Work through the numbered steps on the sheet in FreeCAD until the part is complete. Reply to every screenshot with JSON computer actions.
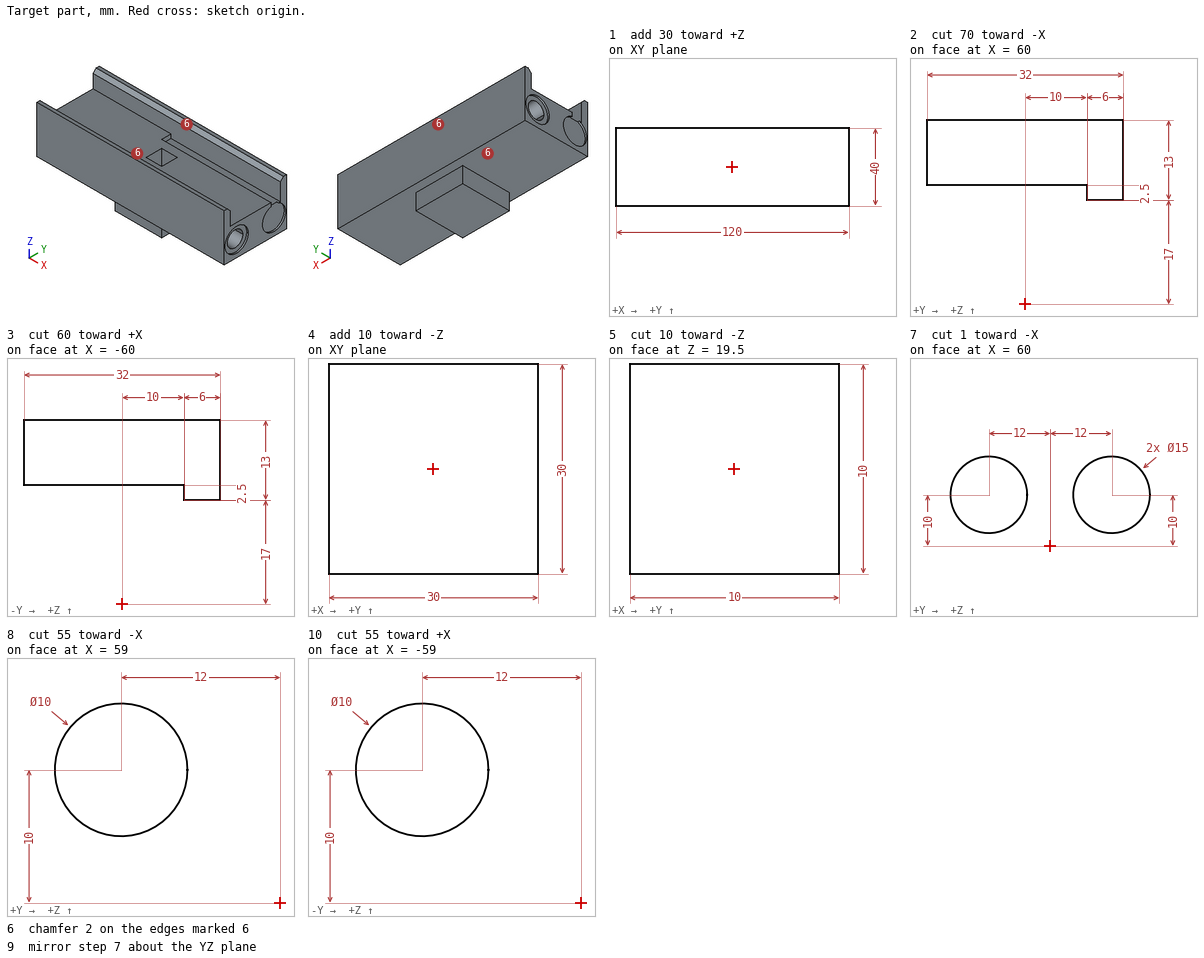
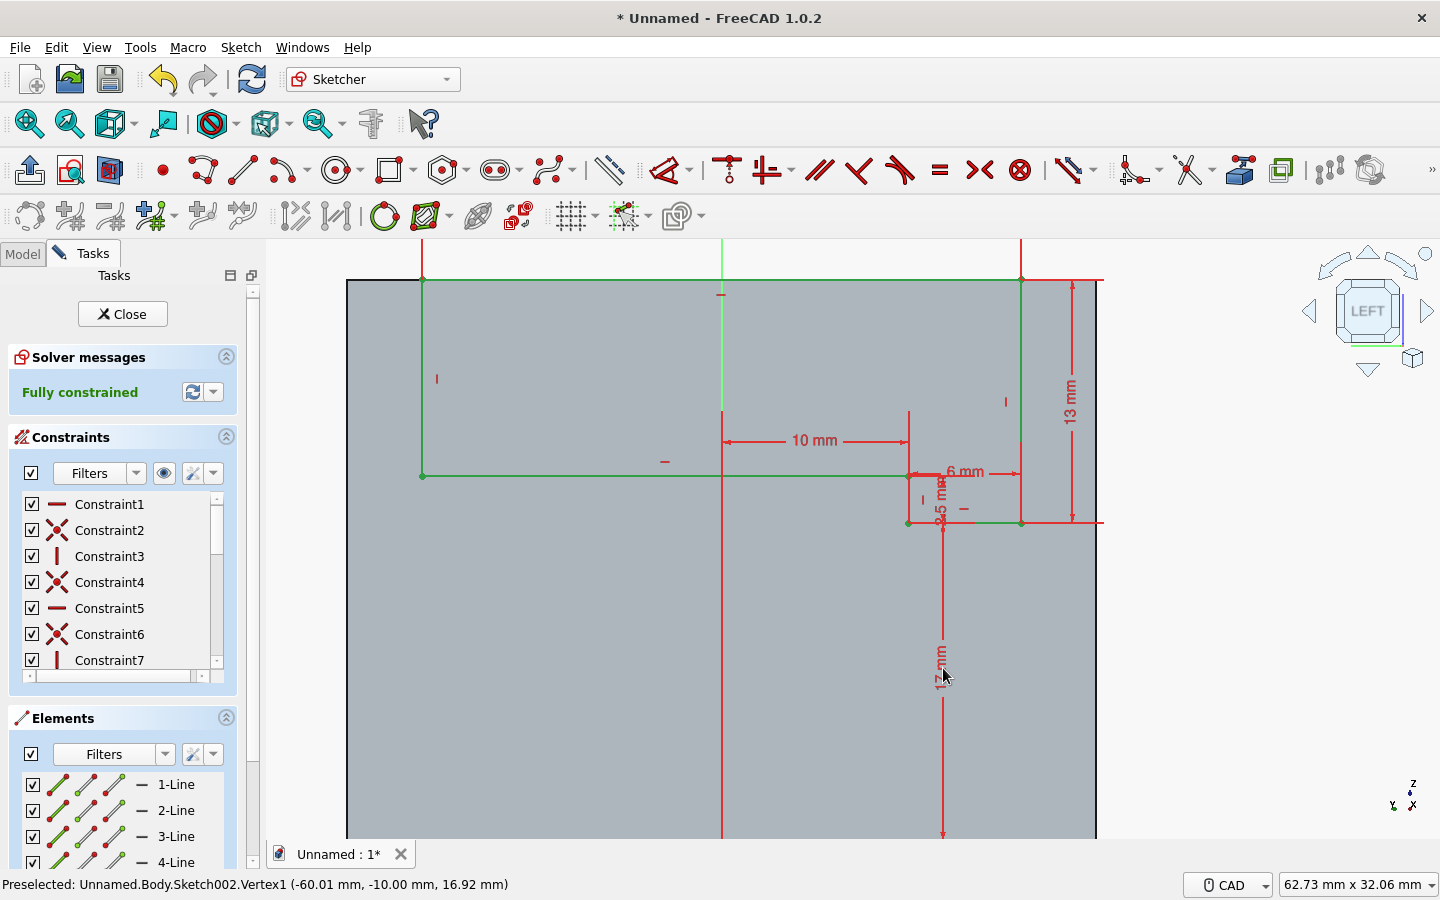
{"action": "left_click", "coordinate": [123, 314]}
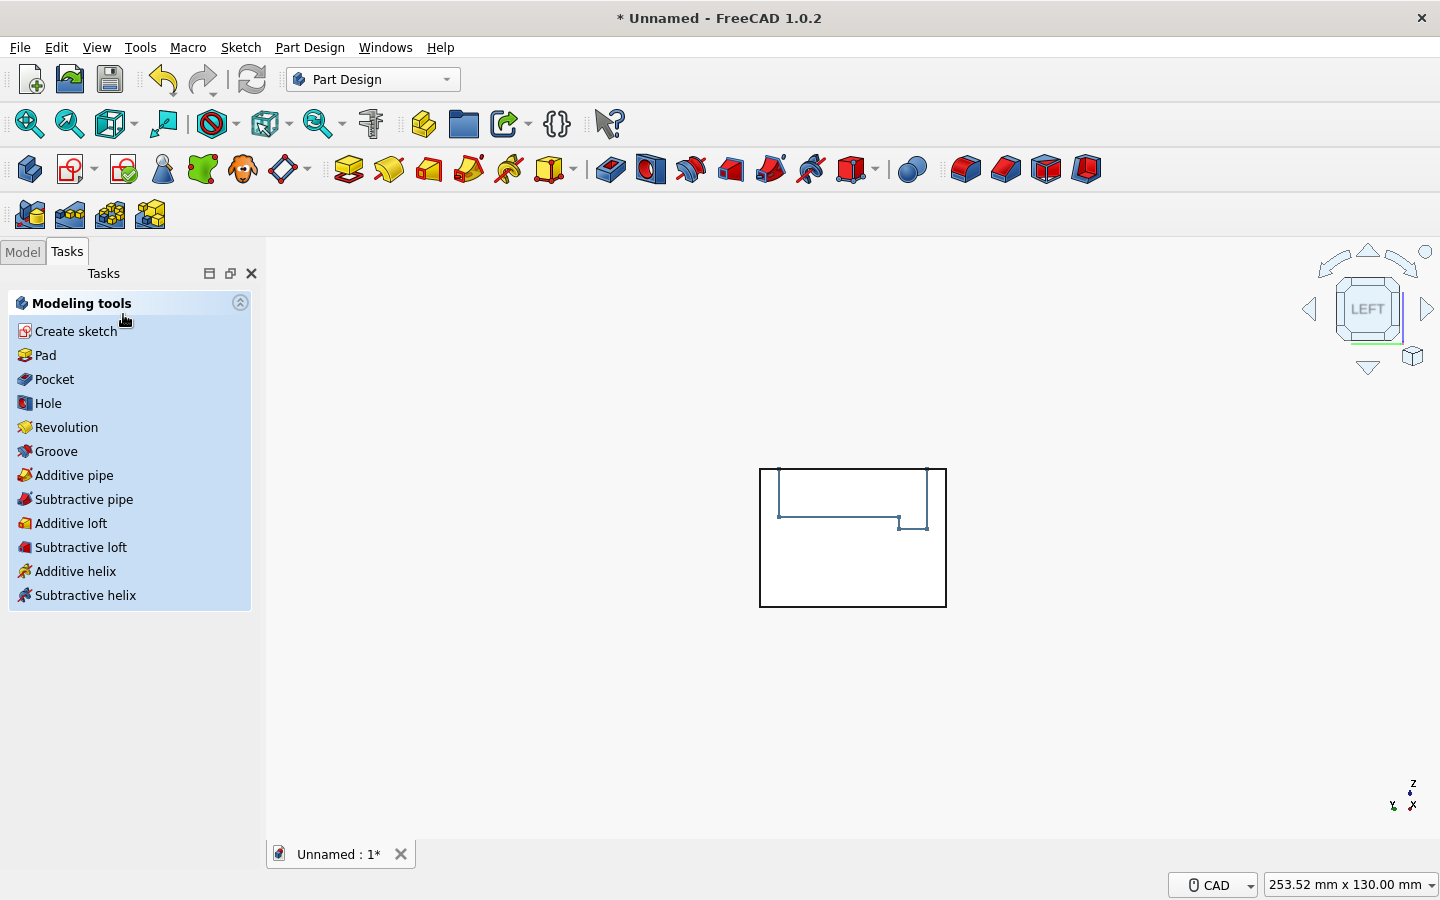
{"action": "left_click", "coordinate": [612, 170]}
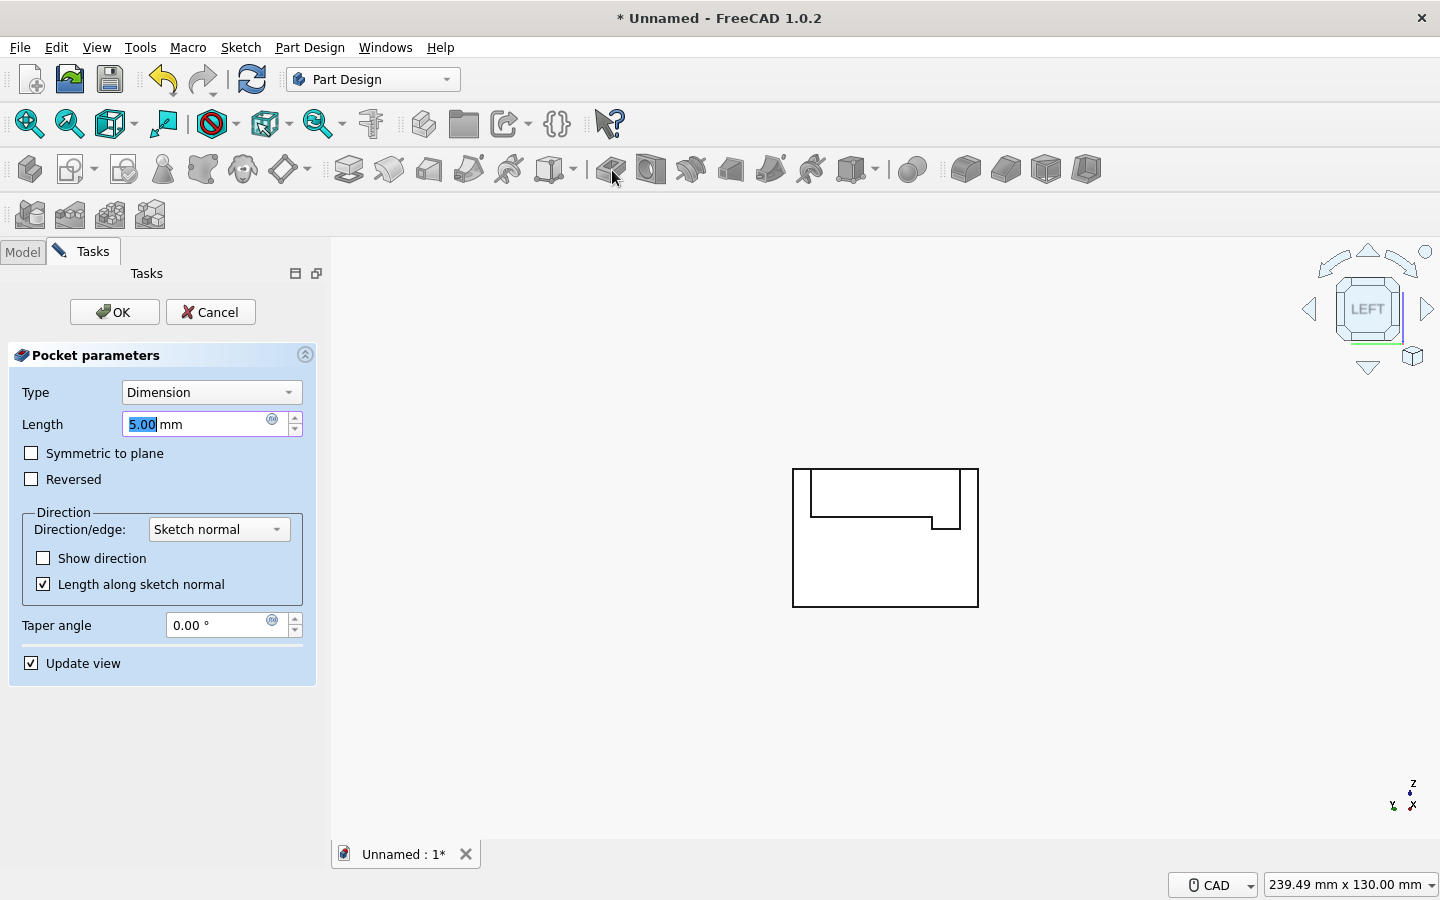
{"action": "type", "text": "60"}
{"action": "key", "text": "Tab"}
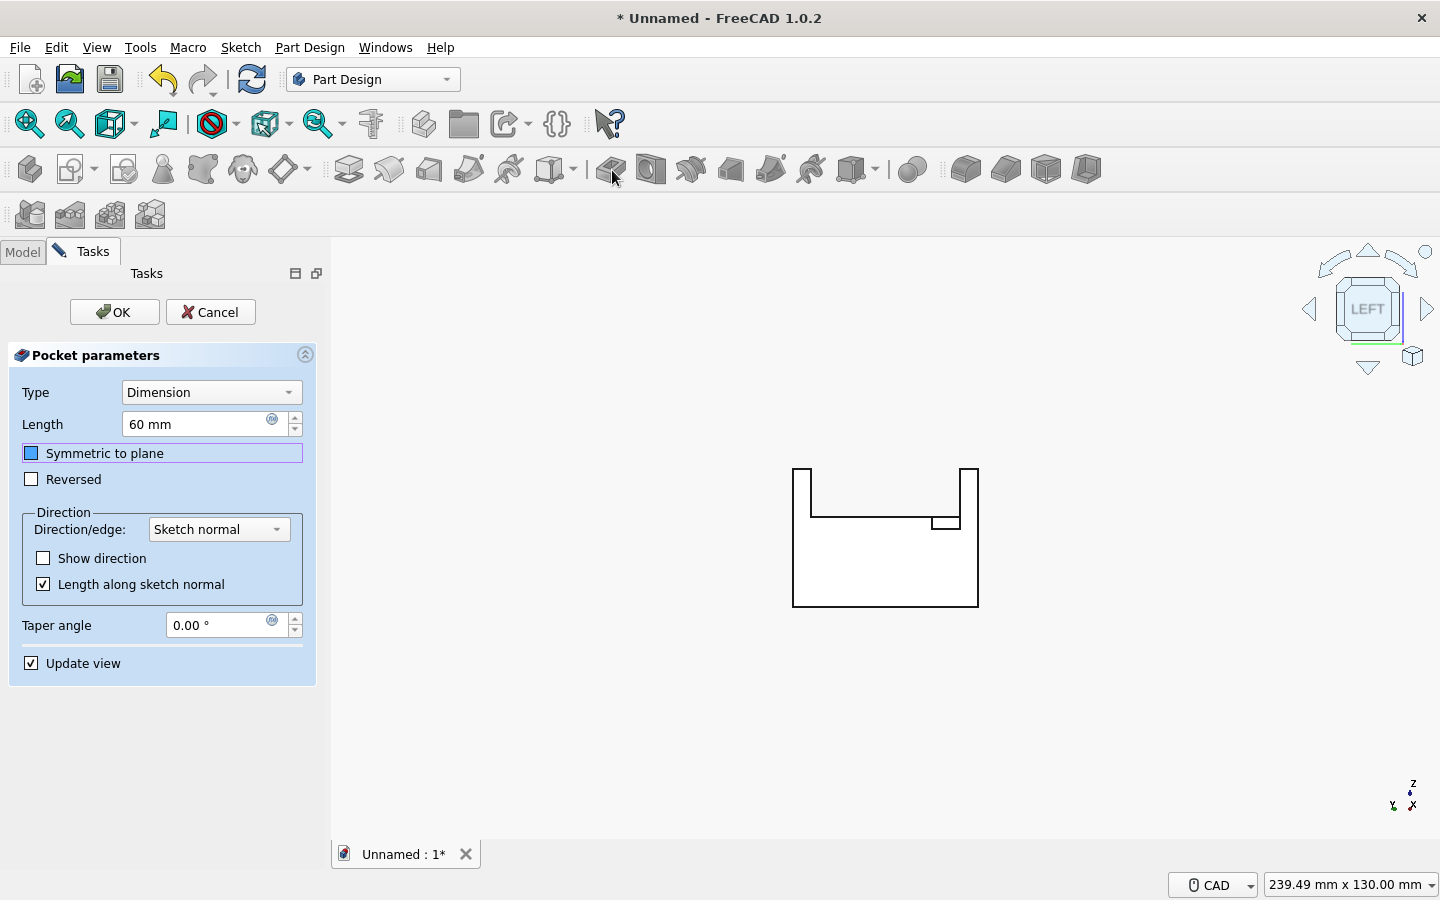
{"action": "left_click", "coordinate": [115, 312]}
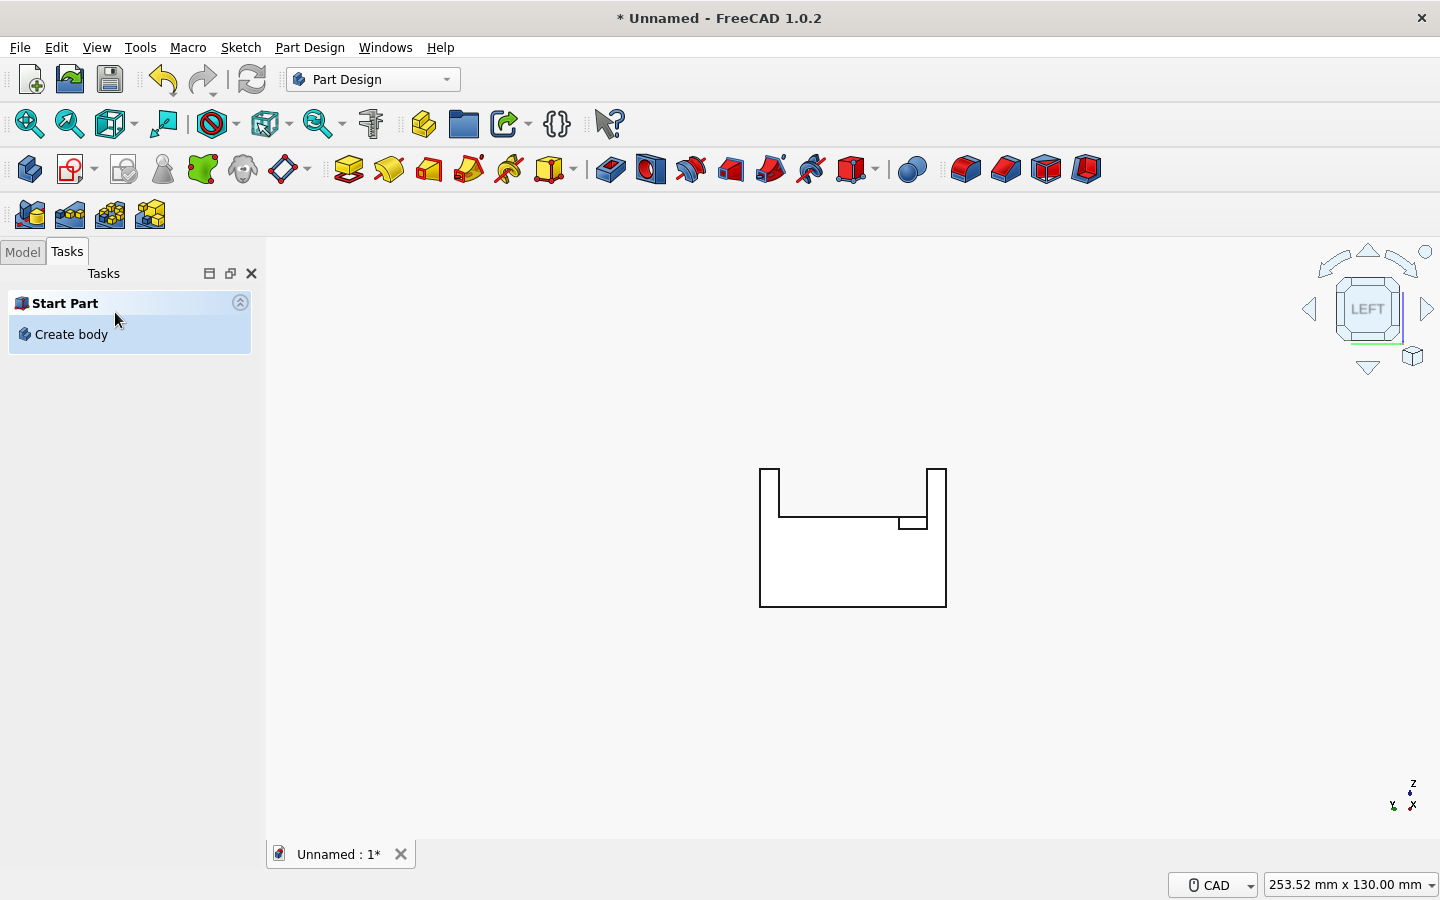
{"action": "left_click", "coordinate": [30, 124]}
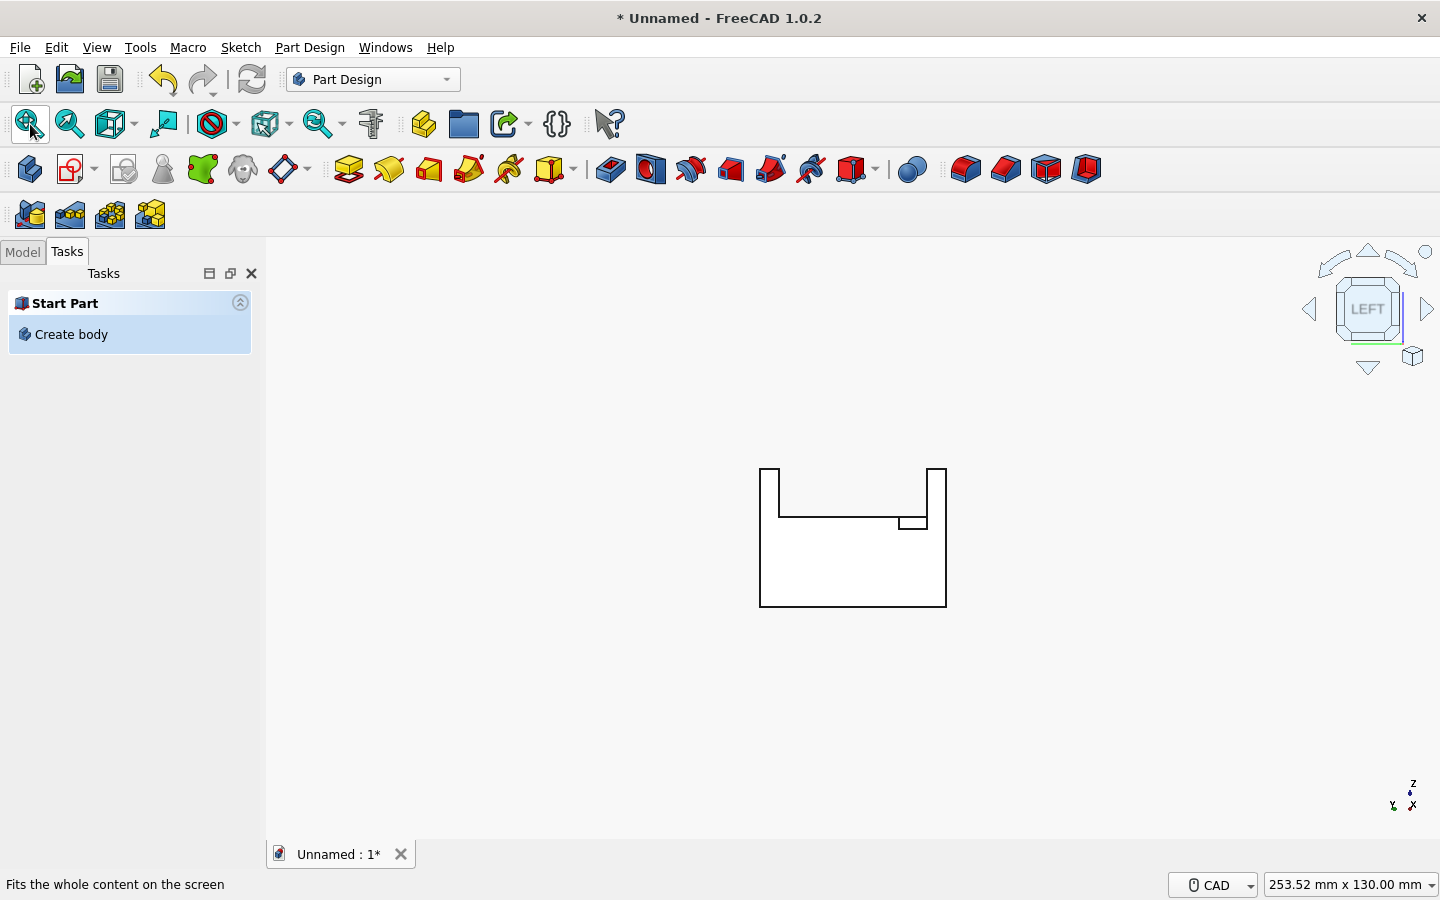
{"action": "left_click", "coordinate": [70, 170]}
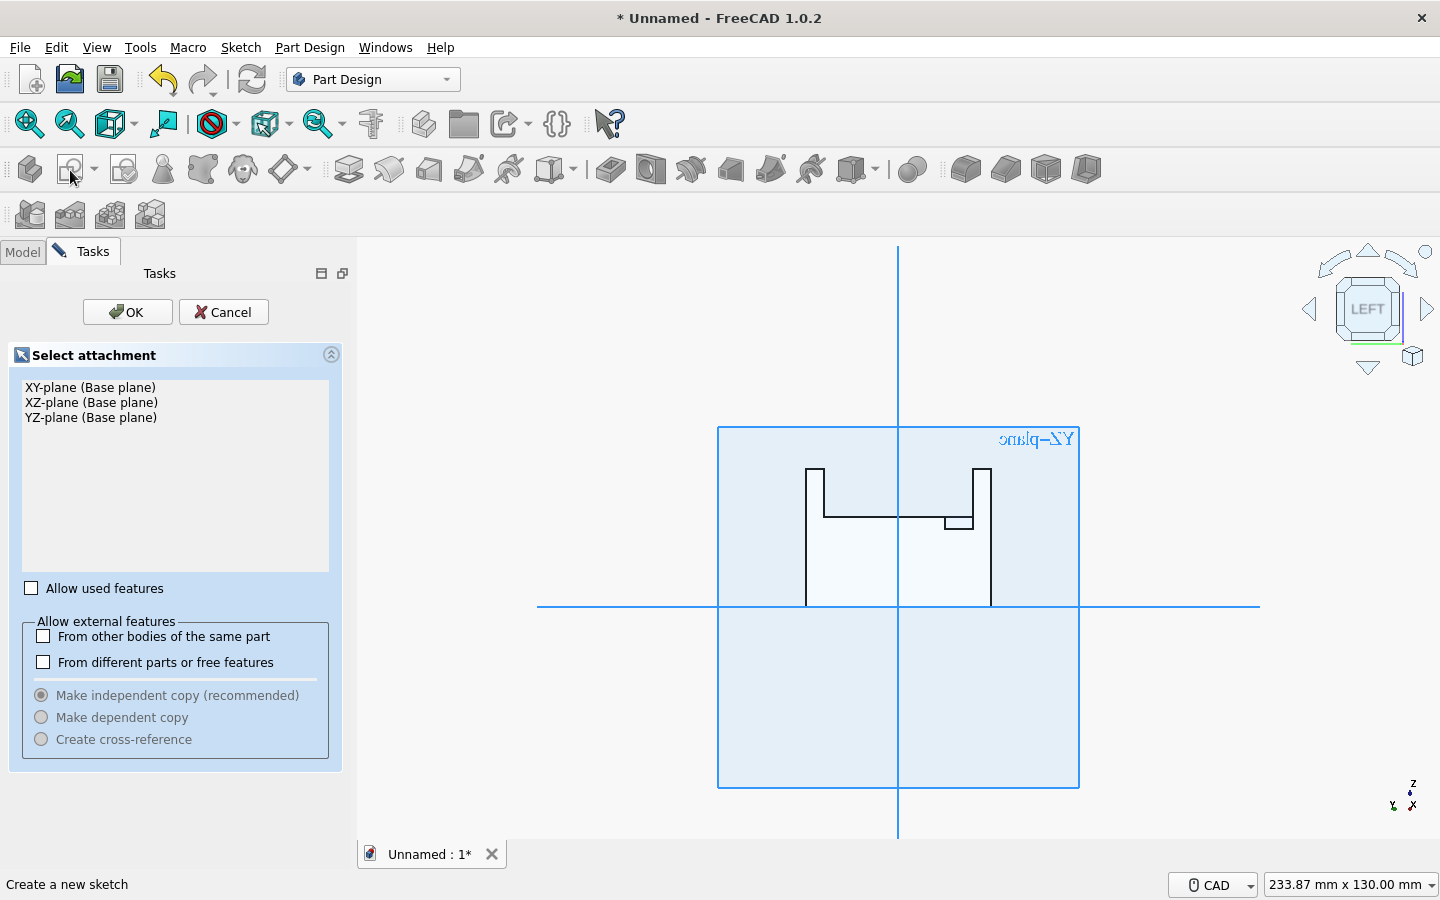
{"action": "left_click", "coordinate": [82, 388]}